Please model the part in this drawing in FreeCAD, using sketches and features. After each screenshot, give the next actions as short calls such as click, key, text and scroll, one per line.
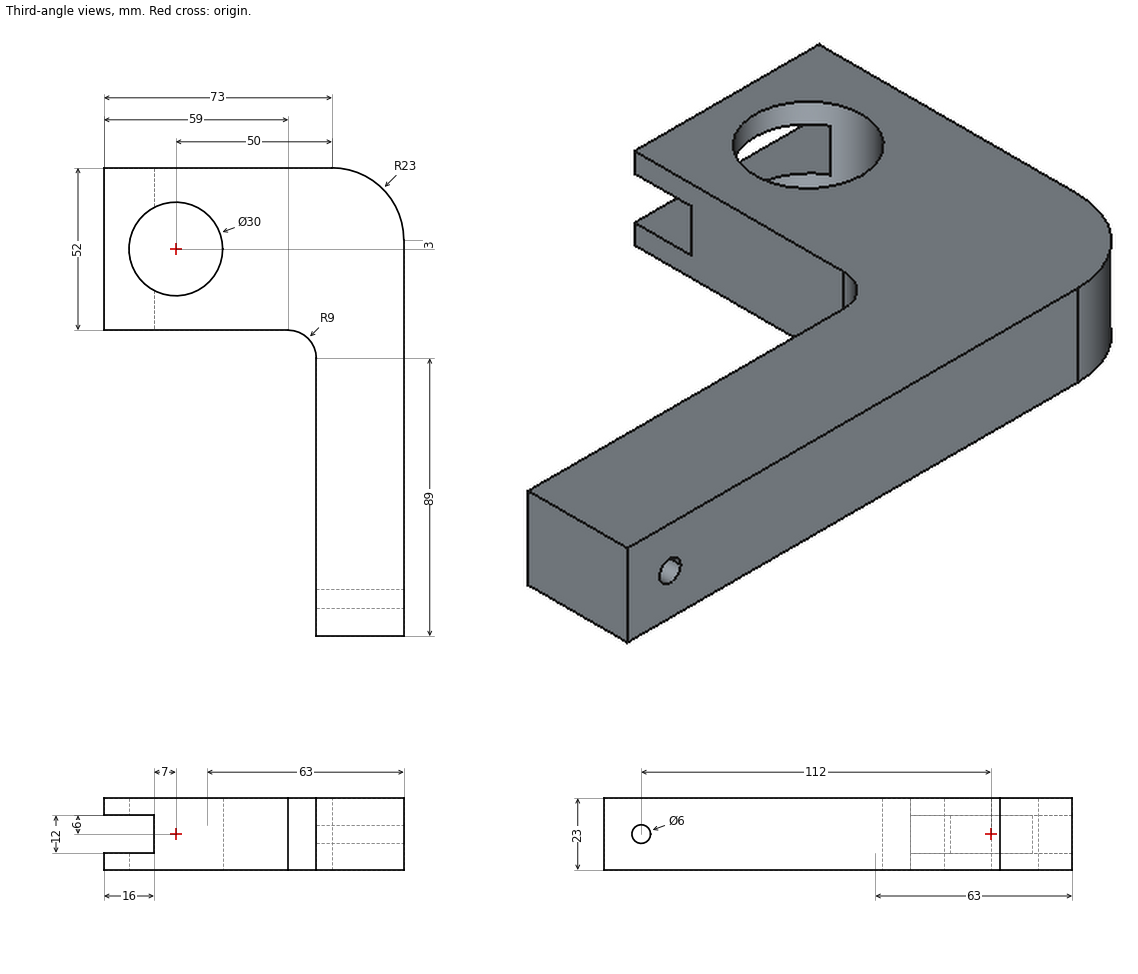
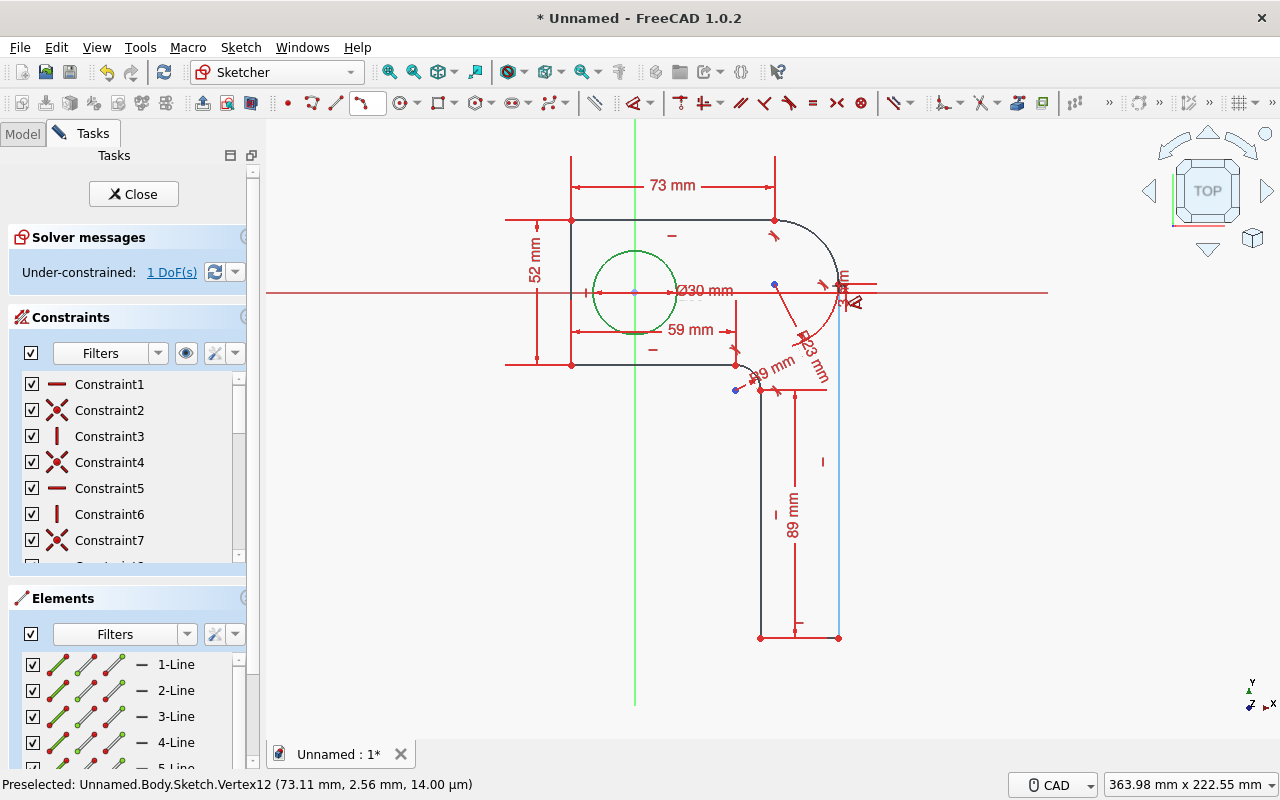
click(775, 220)
click(754, 186)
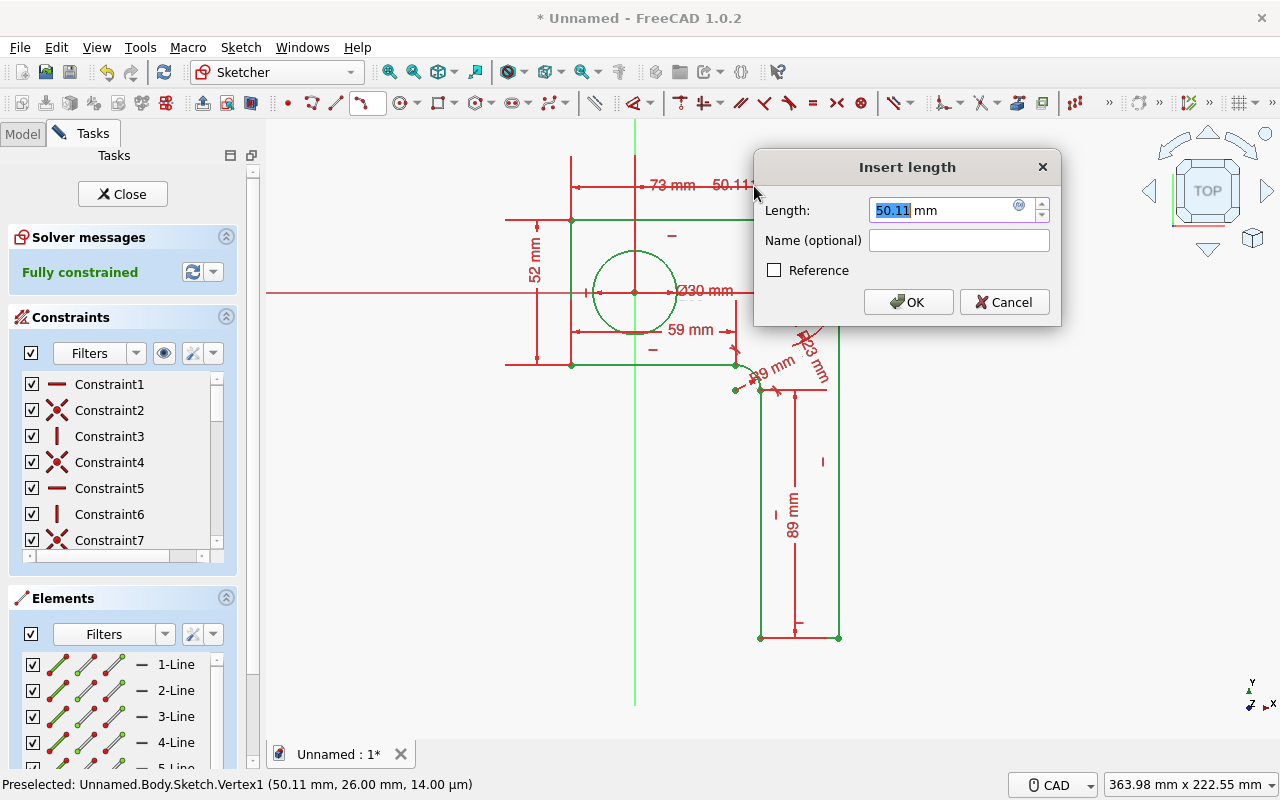
text(50)
key(Return)
key(Escape)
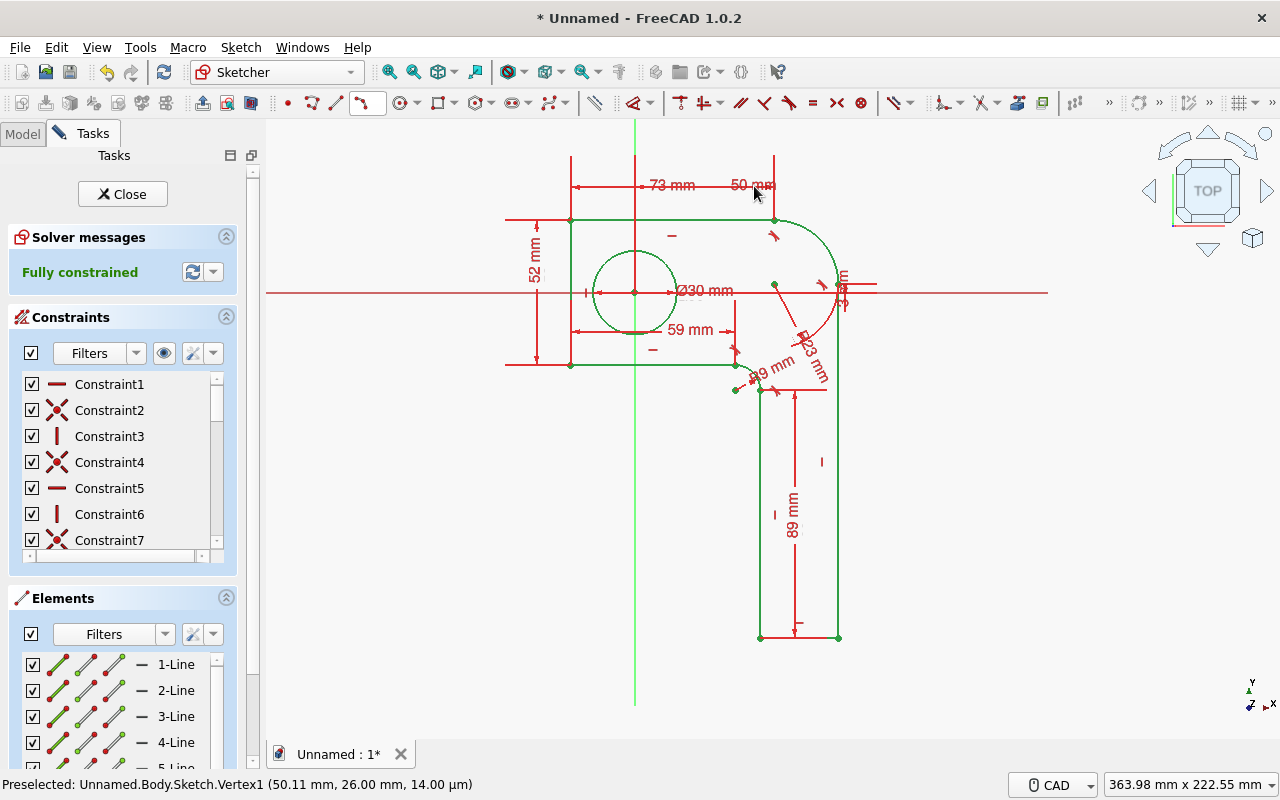
click(123, 194)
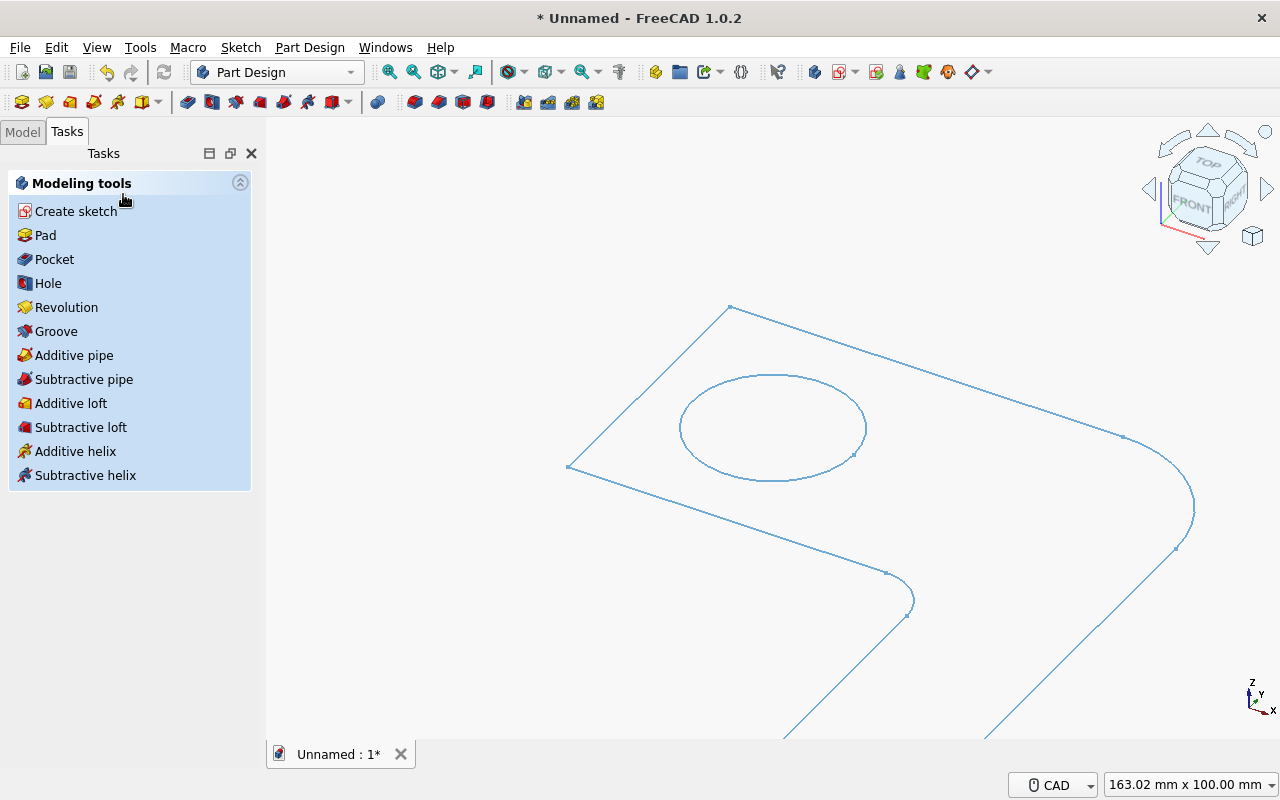
click(22, 102)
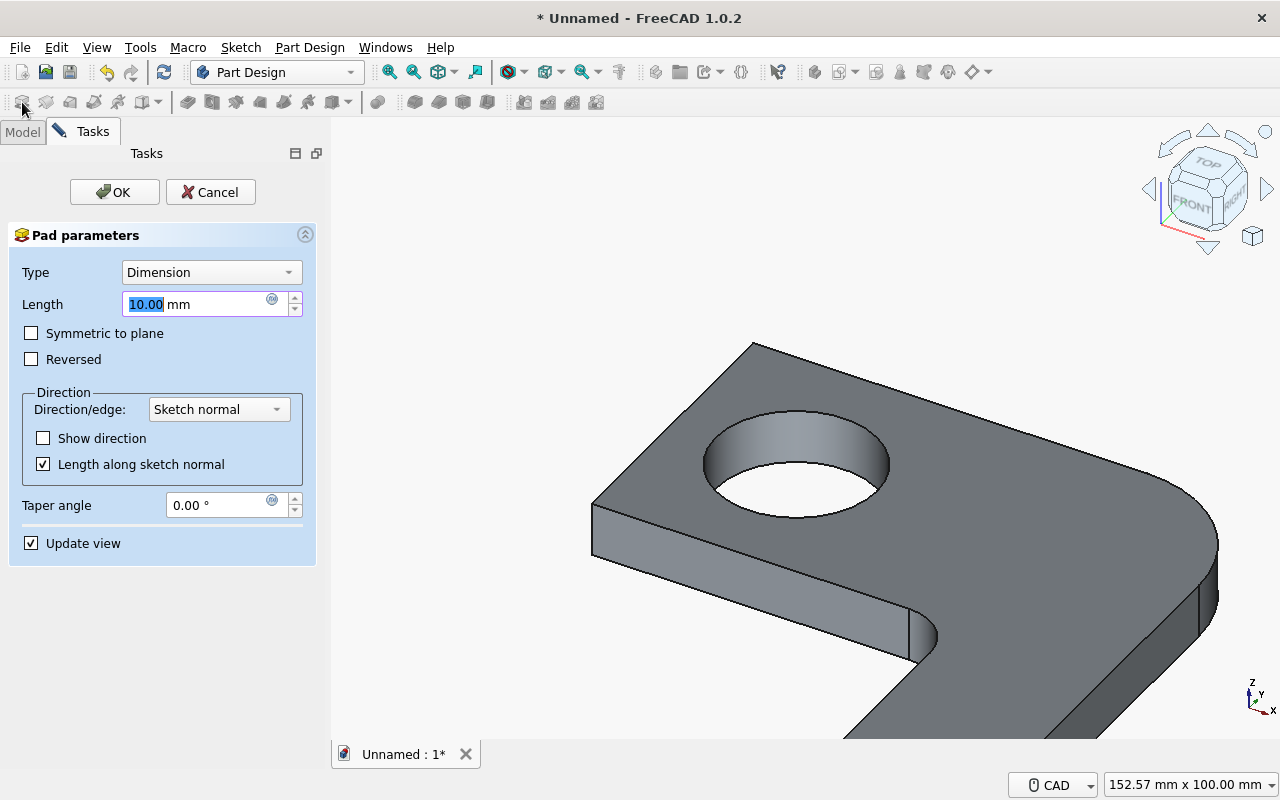
text(23)
key(Tab)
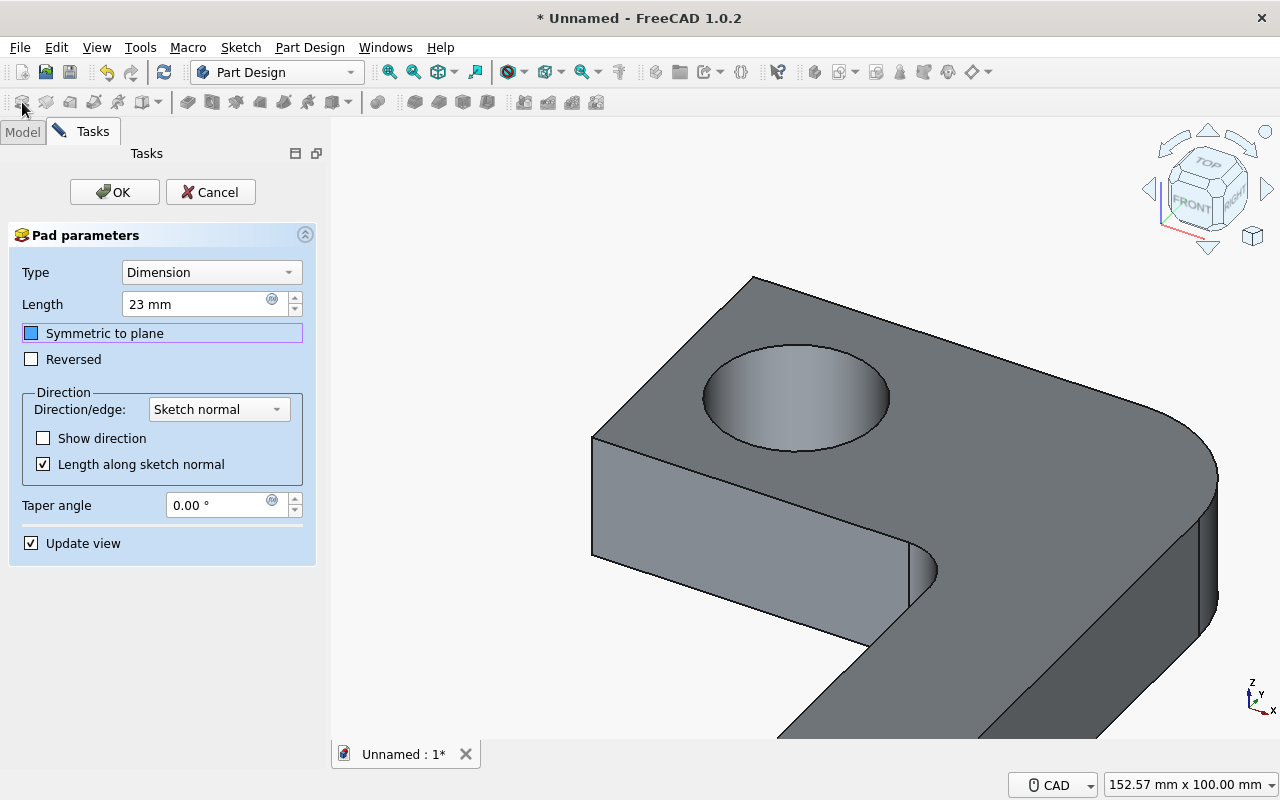
click(30, 333)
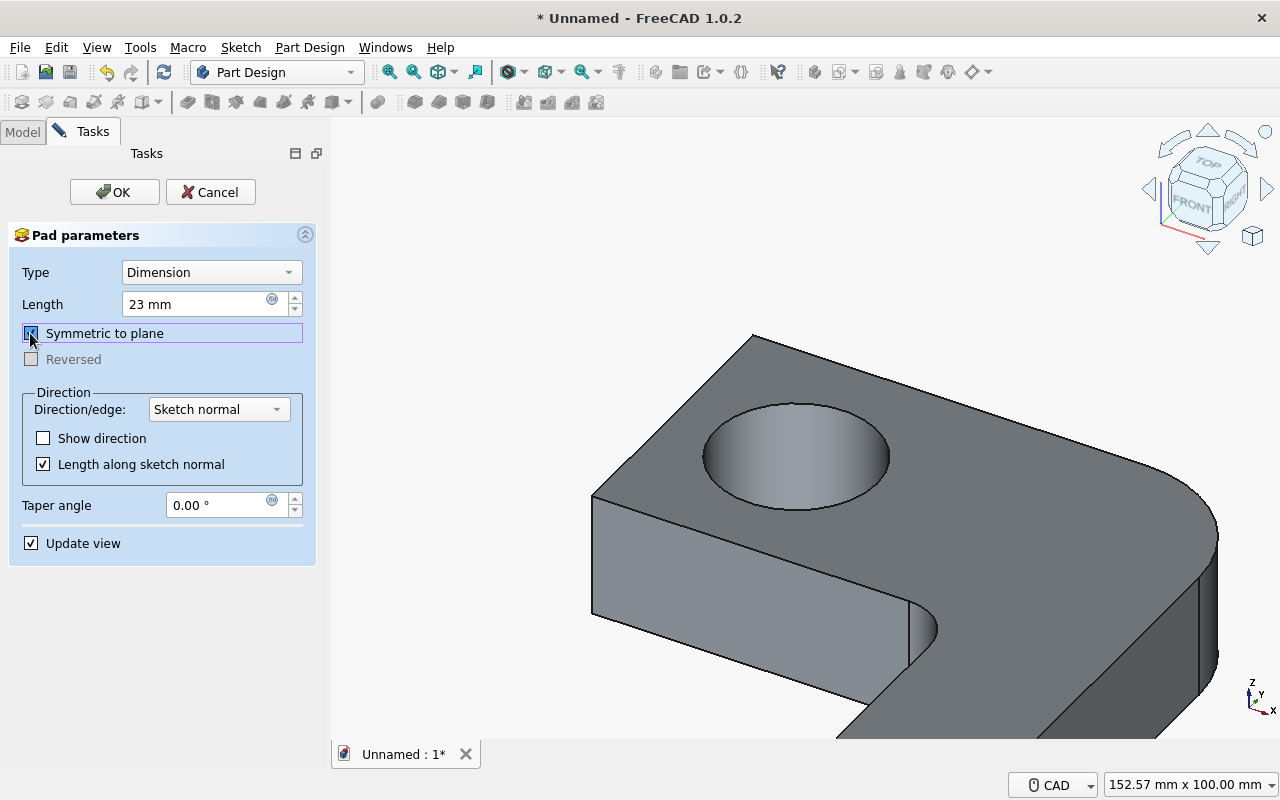
click(115, 192)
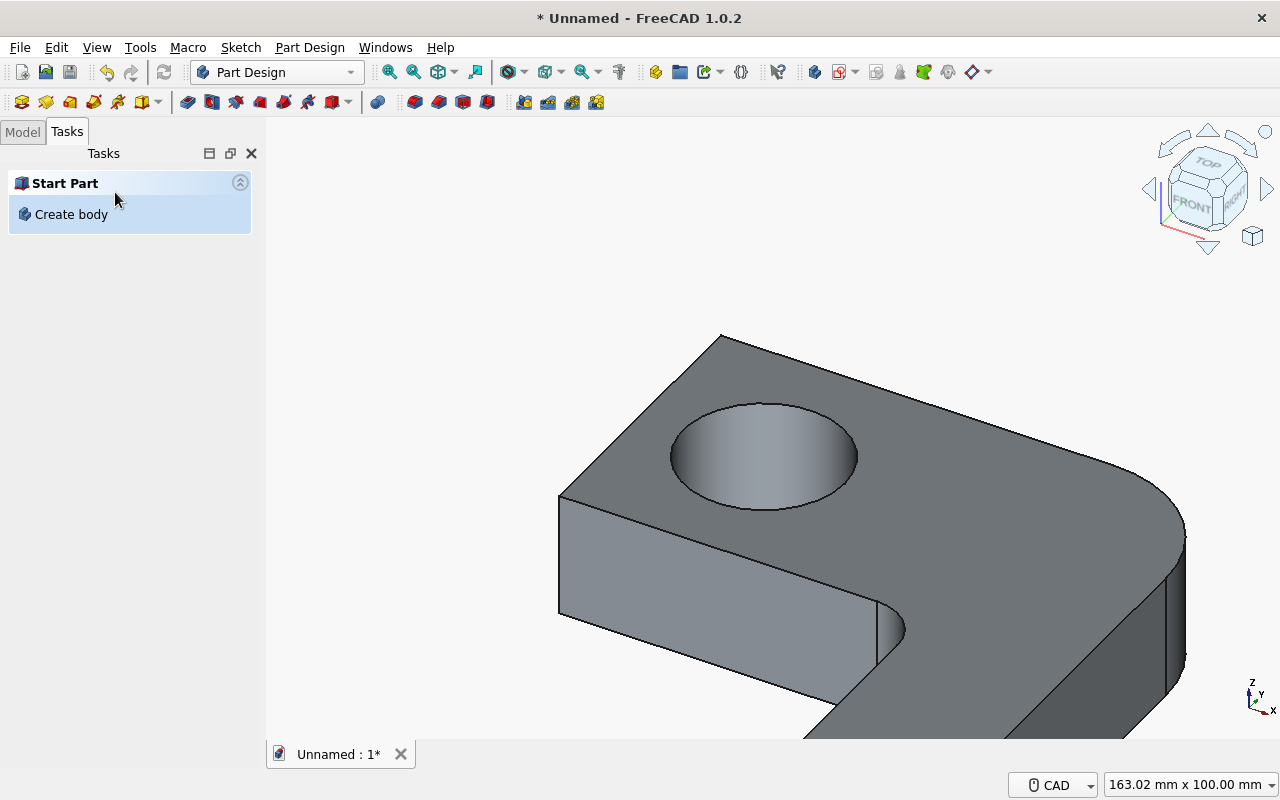
click(390, 72)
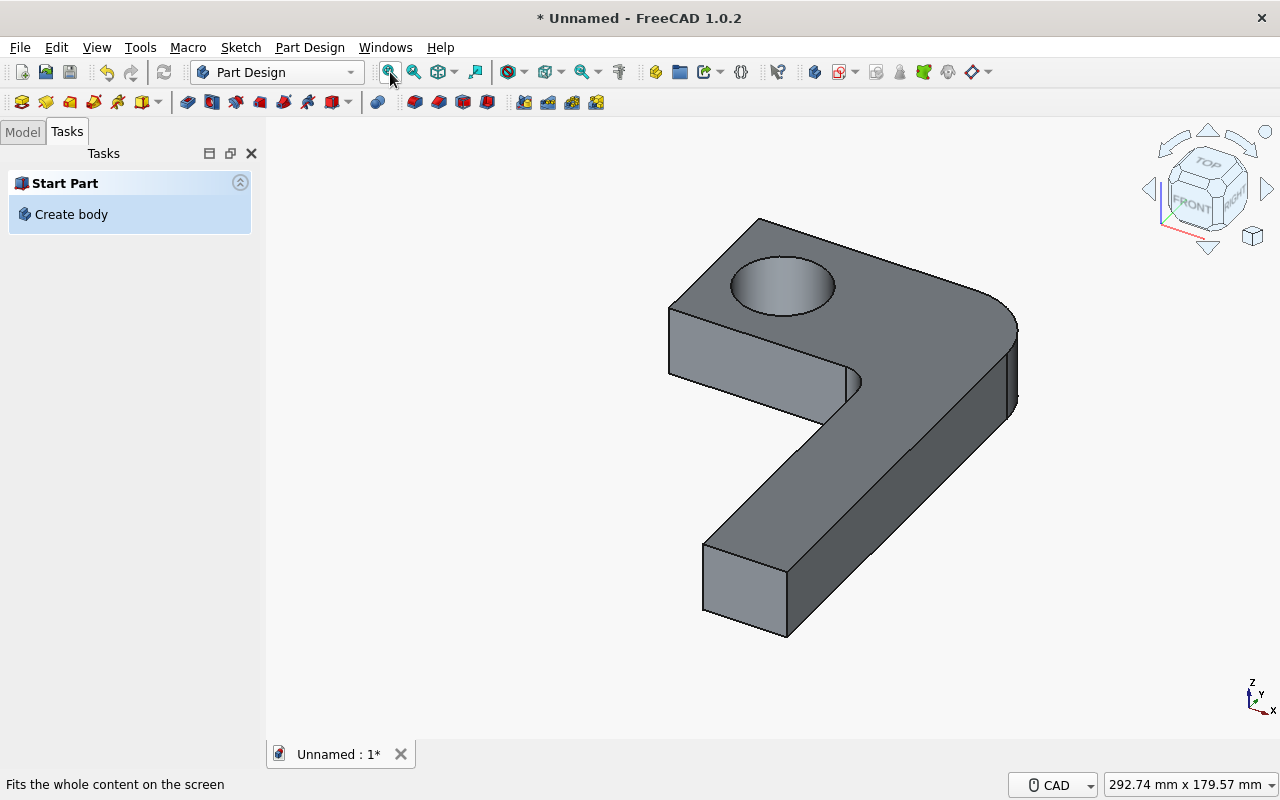
key(4)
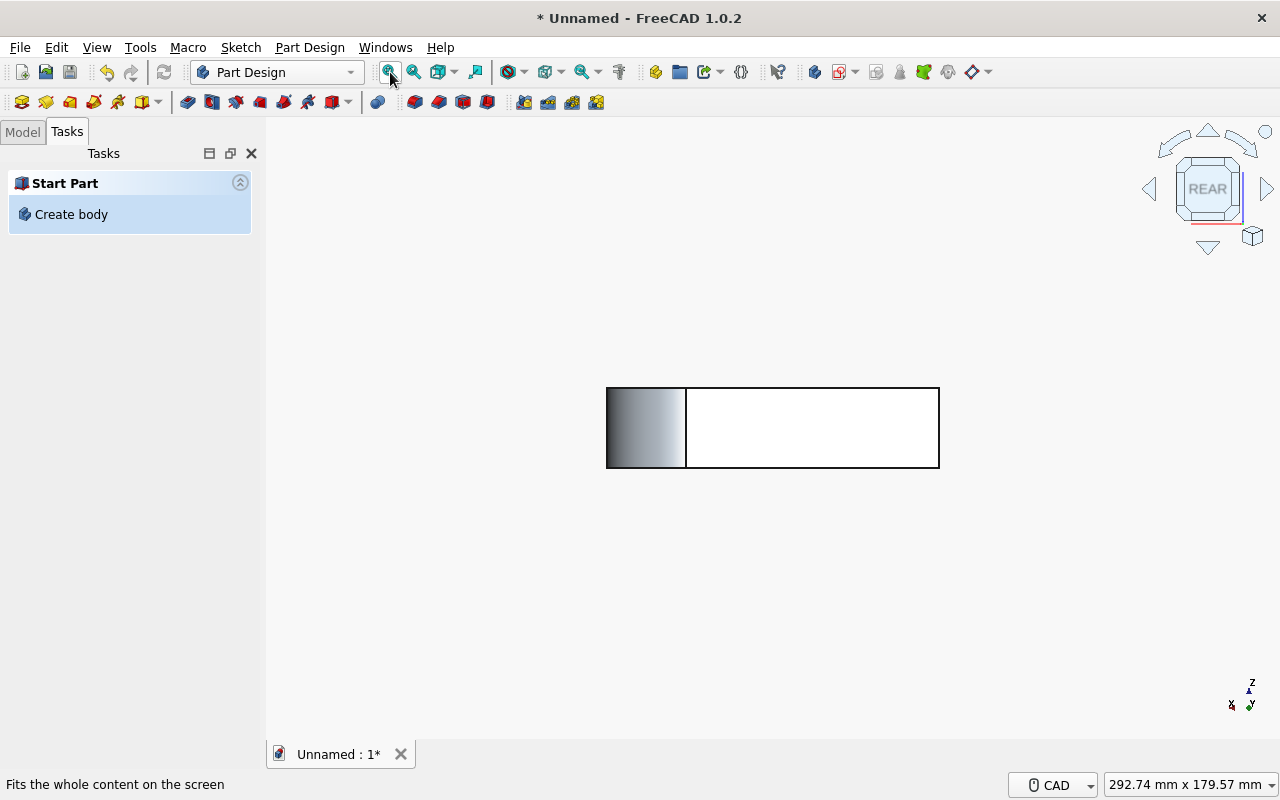
click(390, 72)